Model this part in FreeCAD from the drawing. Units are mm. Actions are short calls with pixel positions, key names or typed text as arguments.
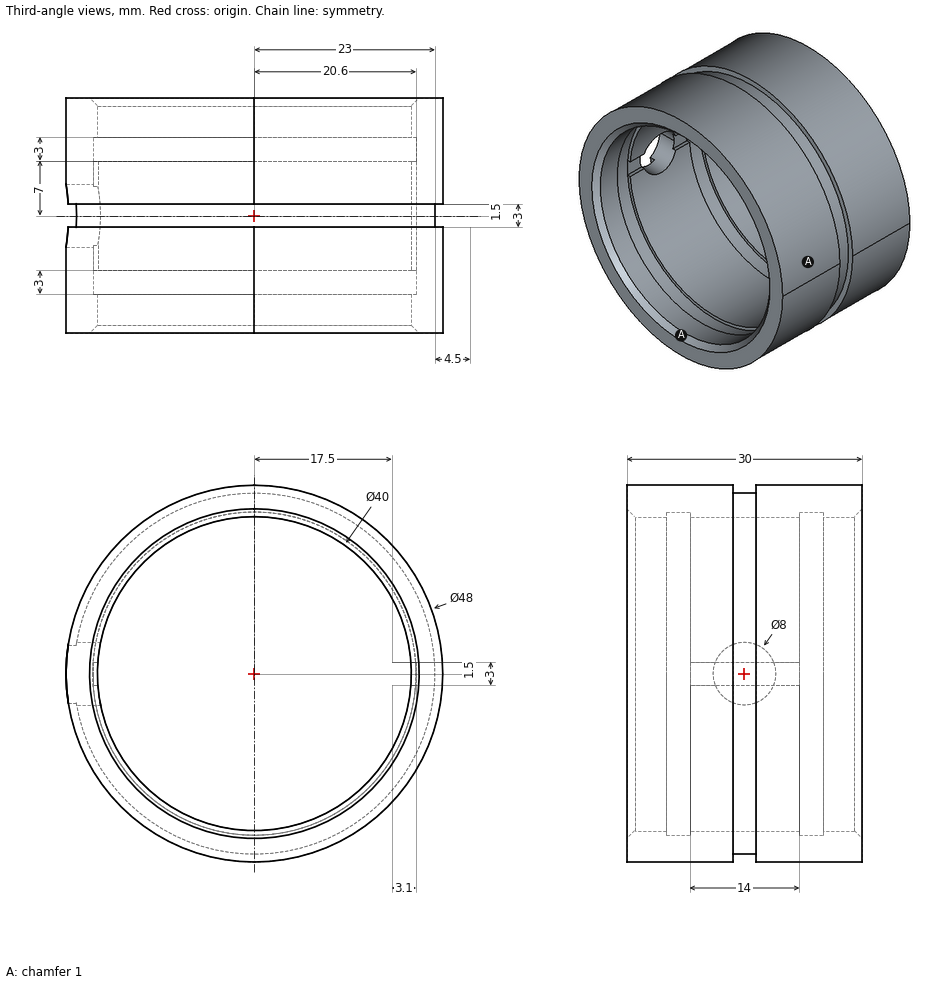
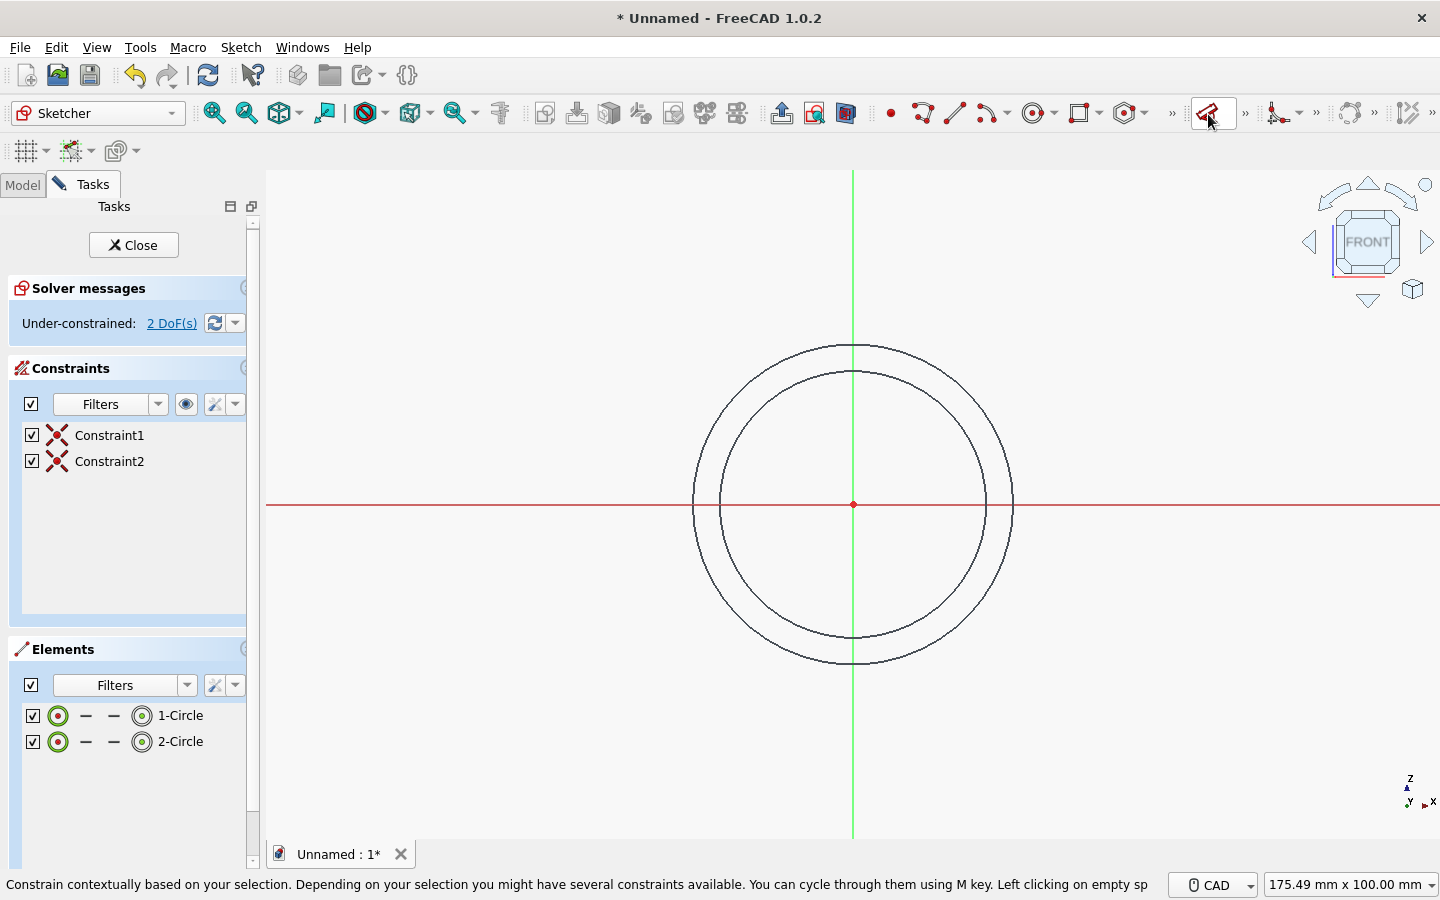
click(966, 391)
click(989, 368)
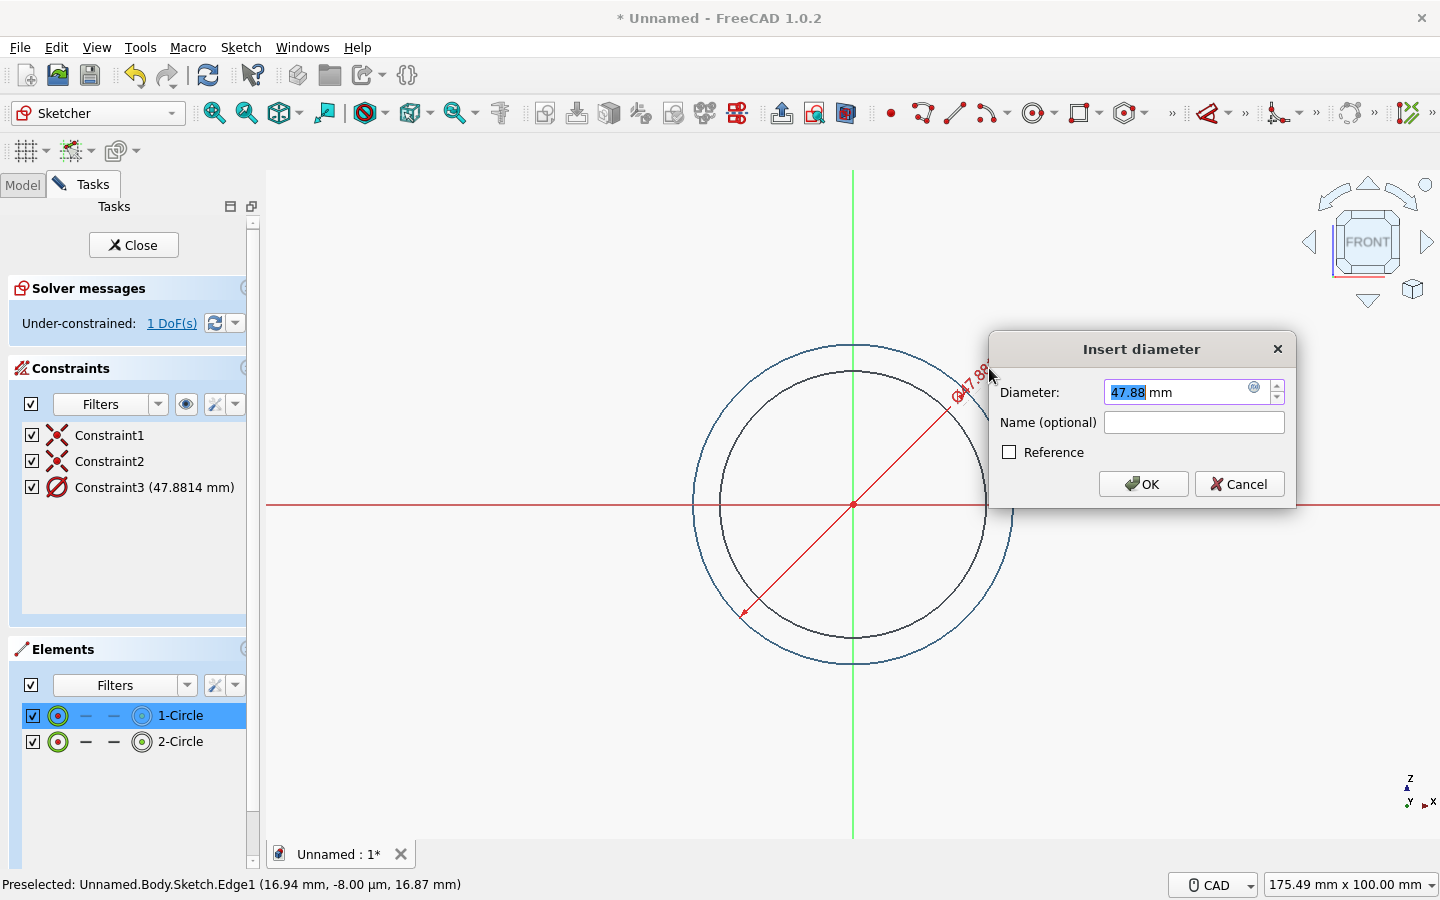
text(48)
key(Return)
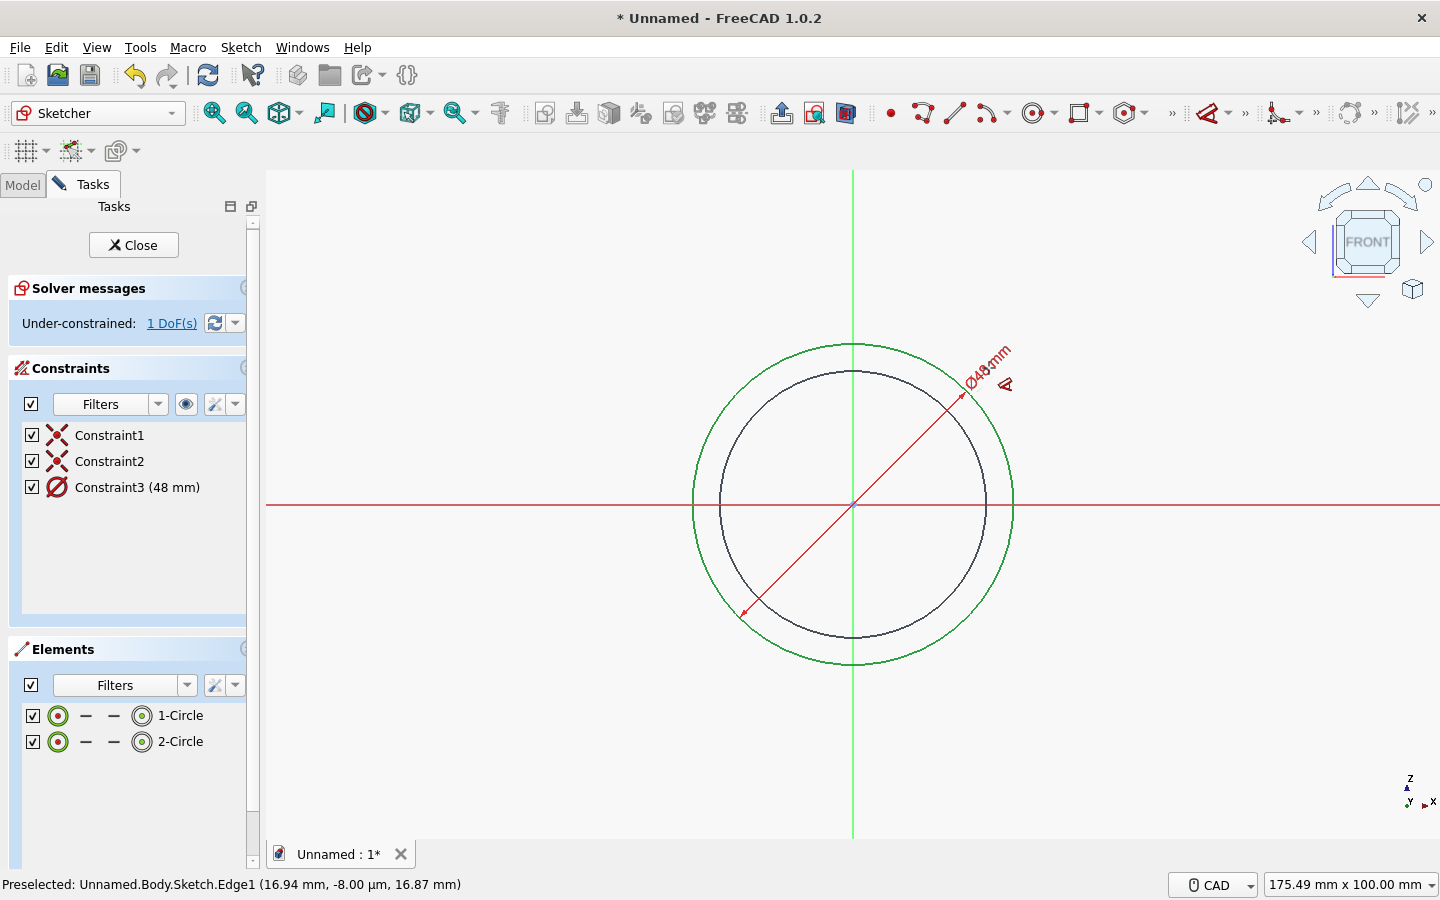
click(947, 410)
click(1034, 451)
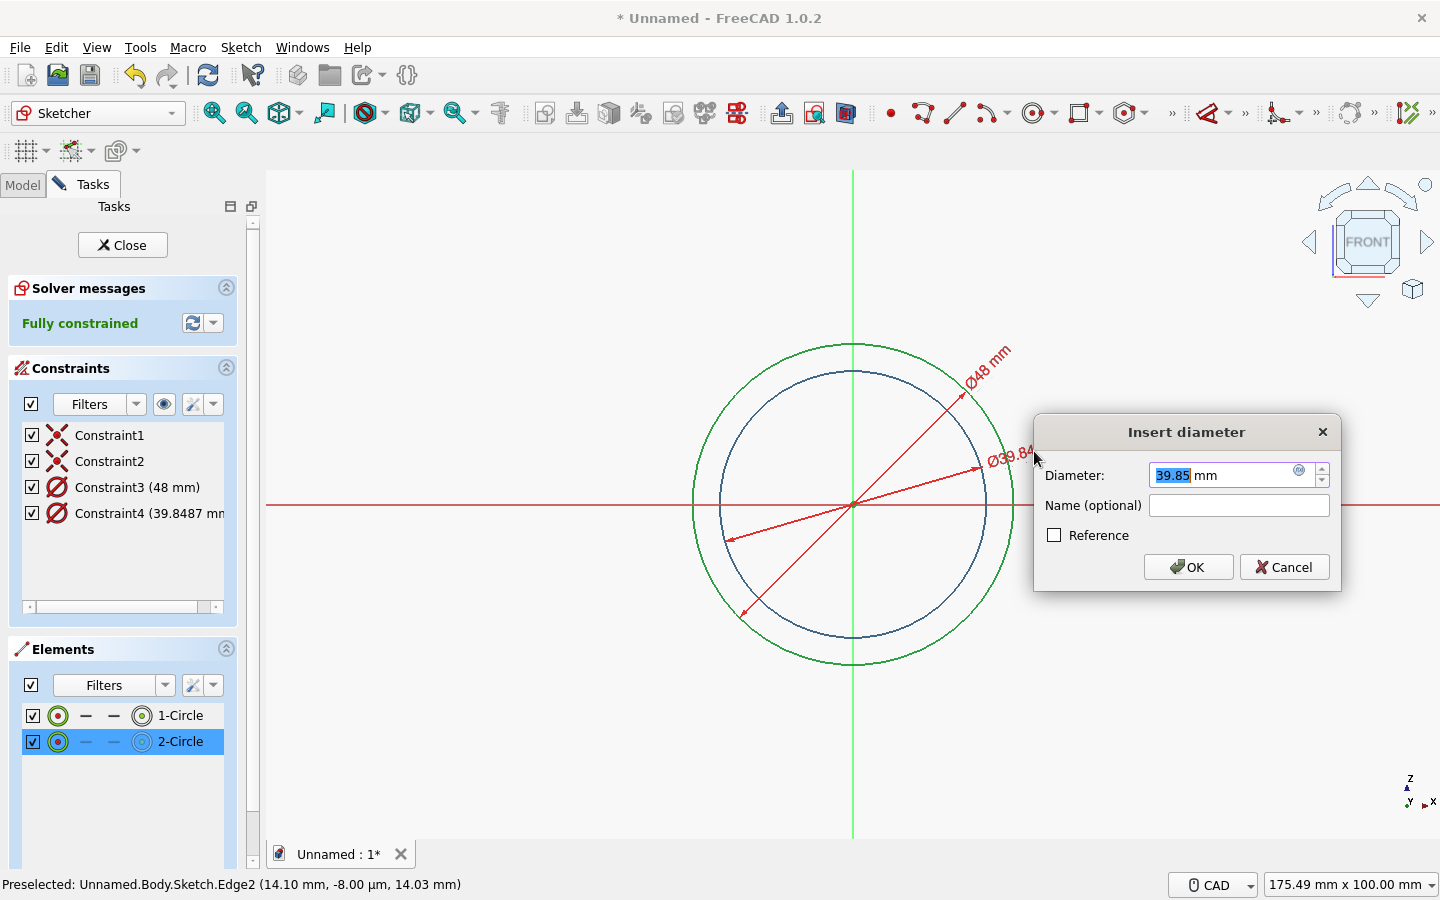
text(40)
key(Return)
key(Escape)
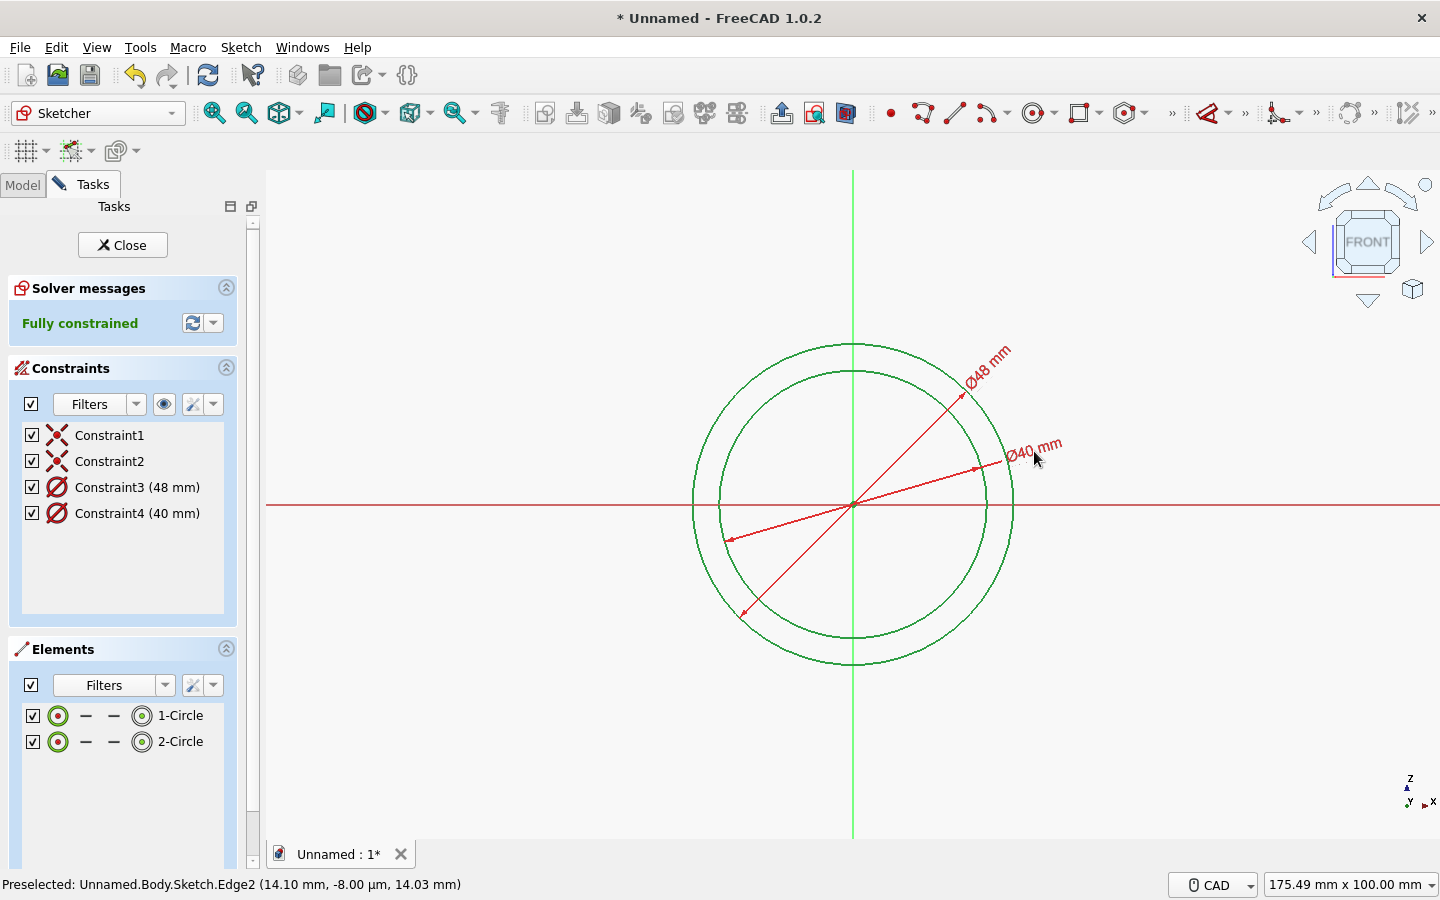
click(123, 245)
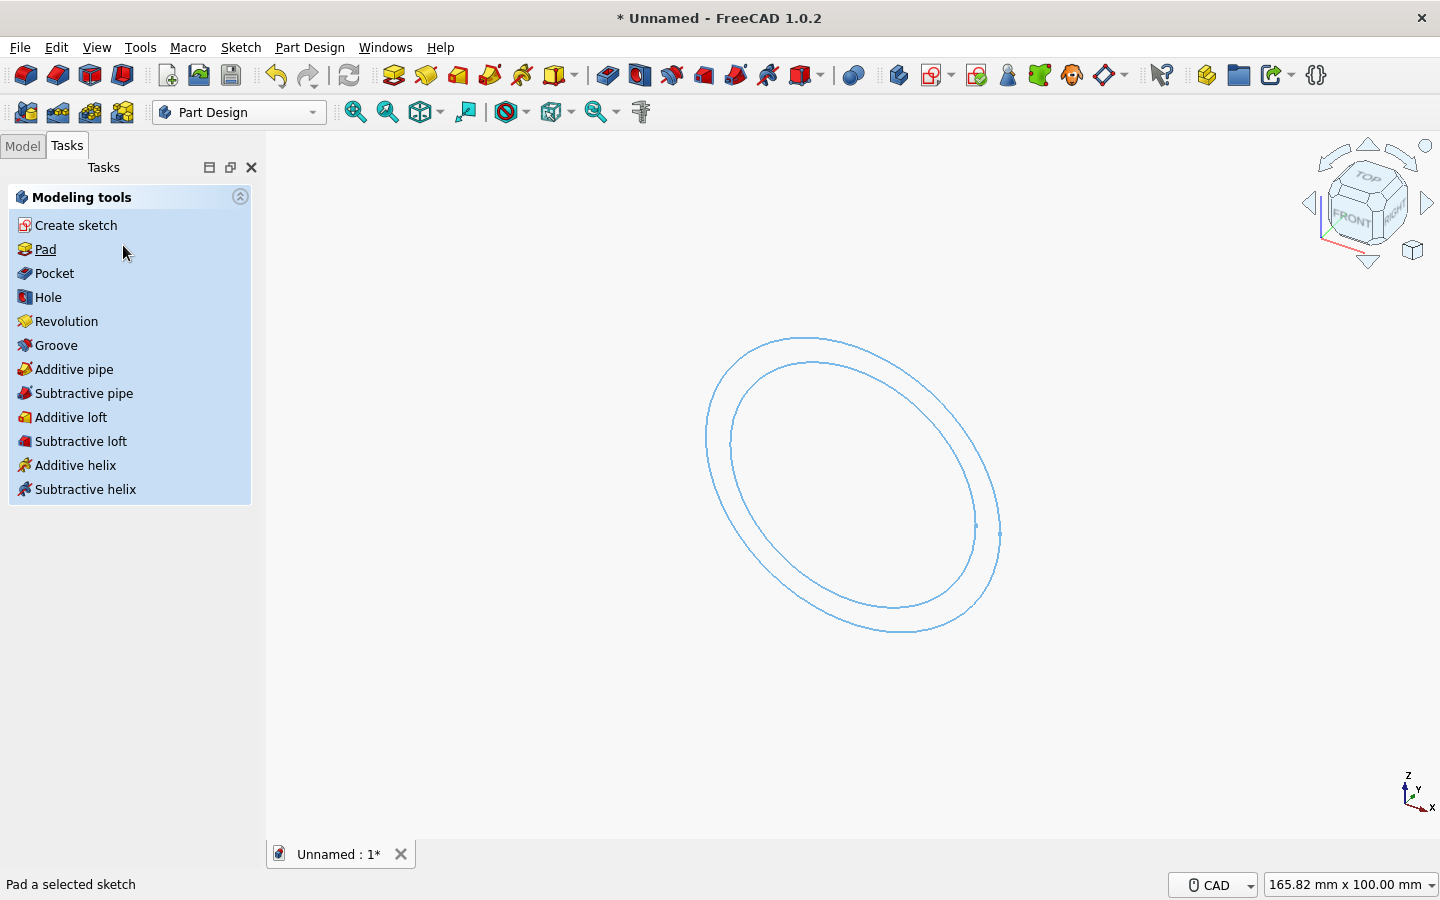
click(394, 76)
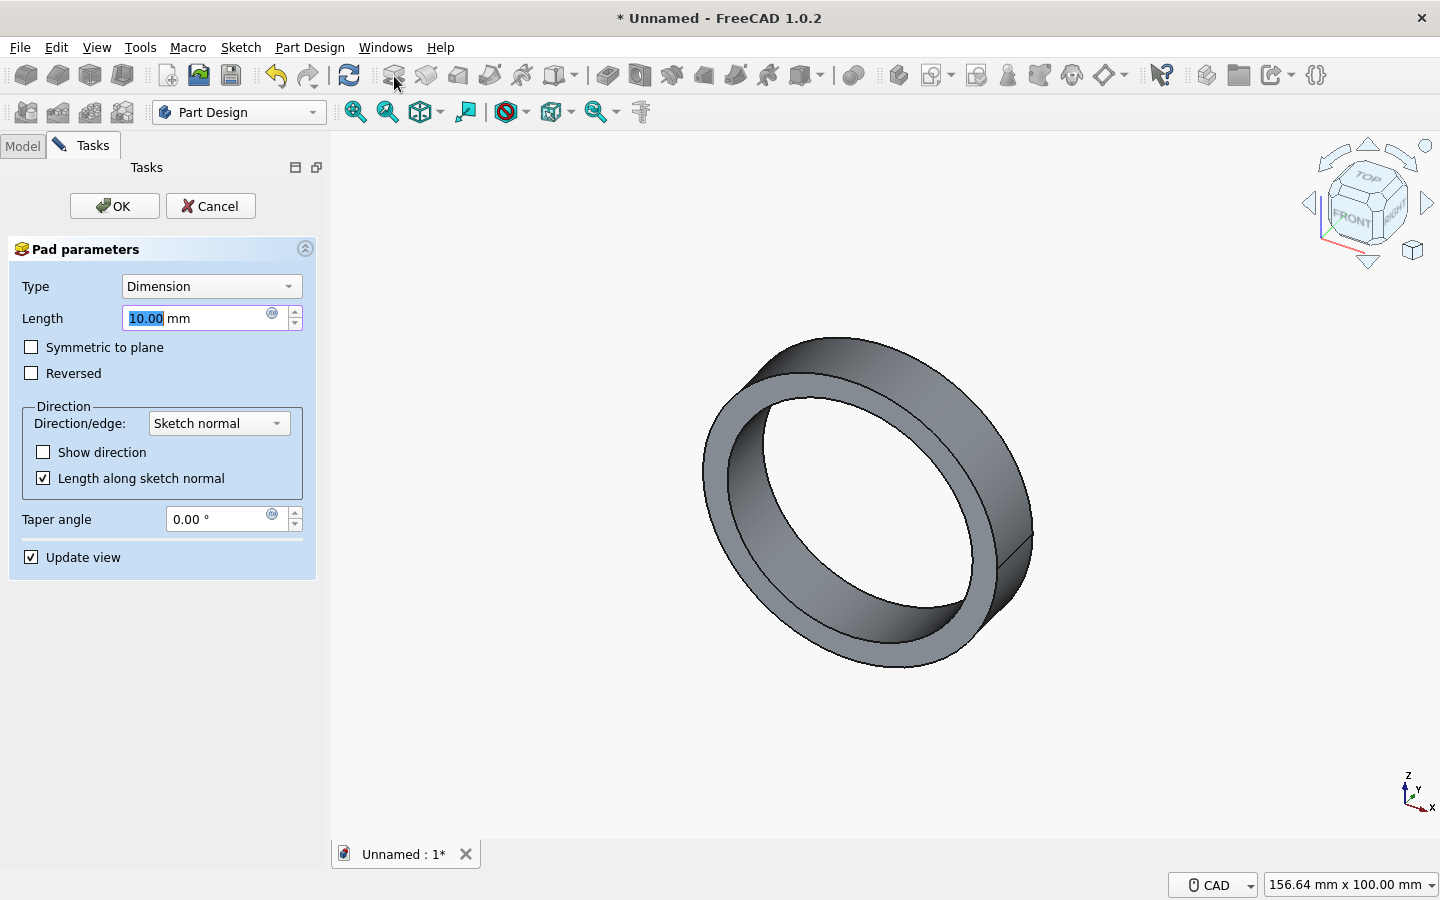
text(30)
key(Tab)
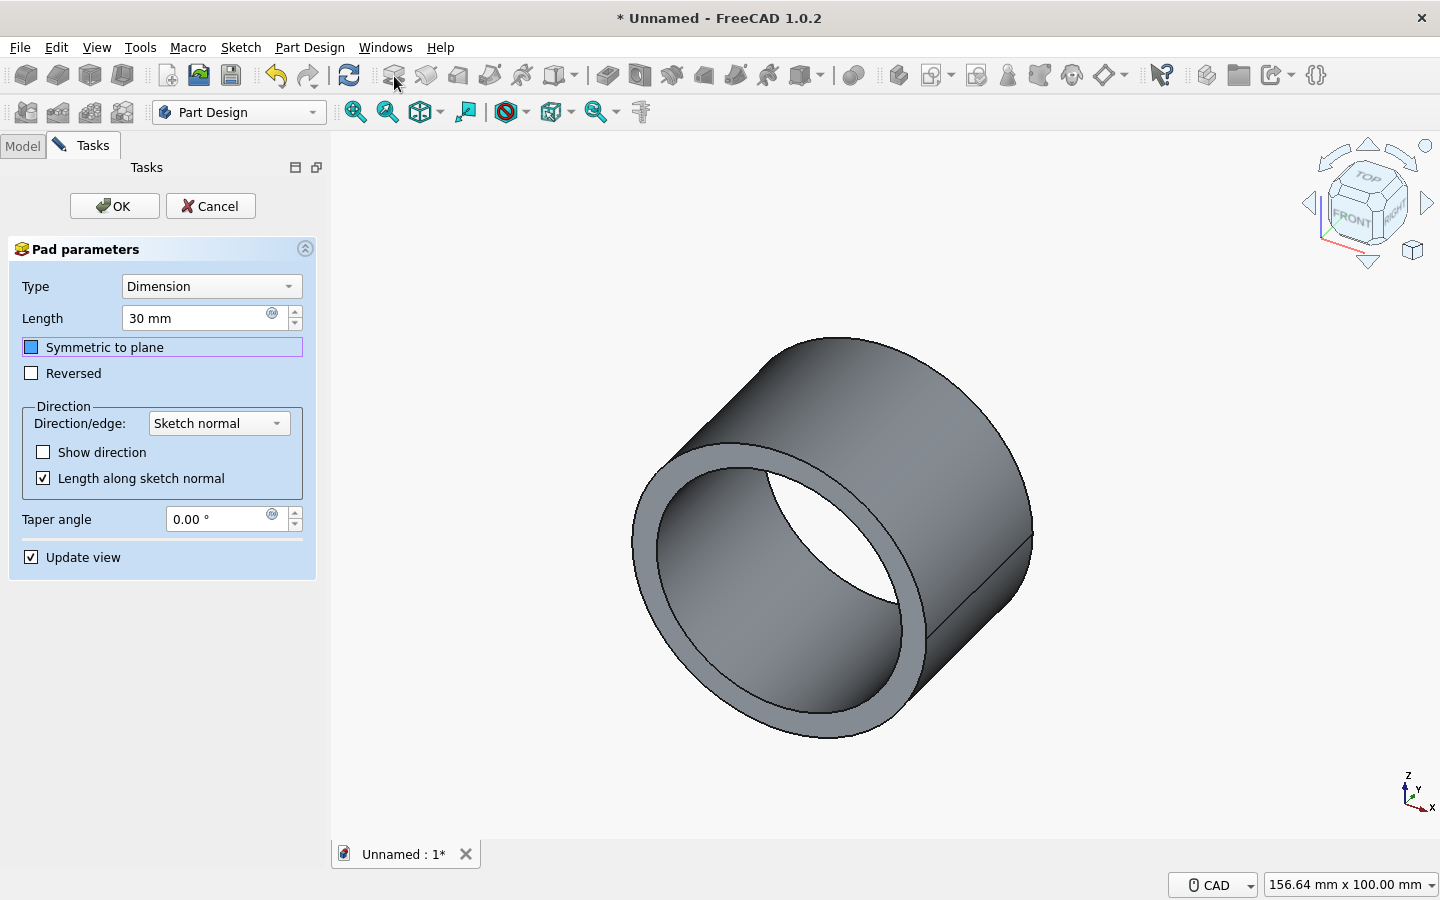
click(30, 347)